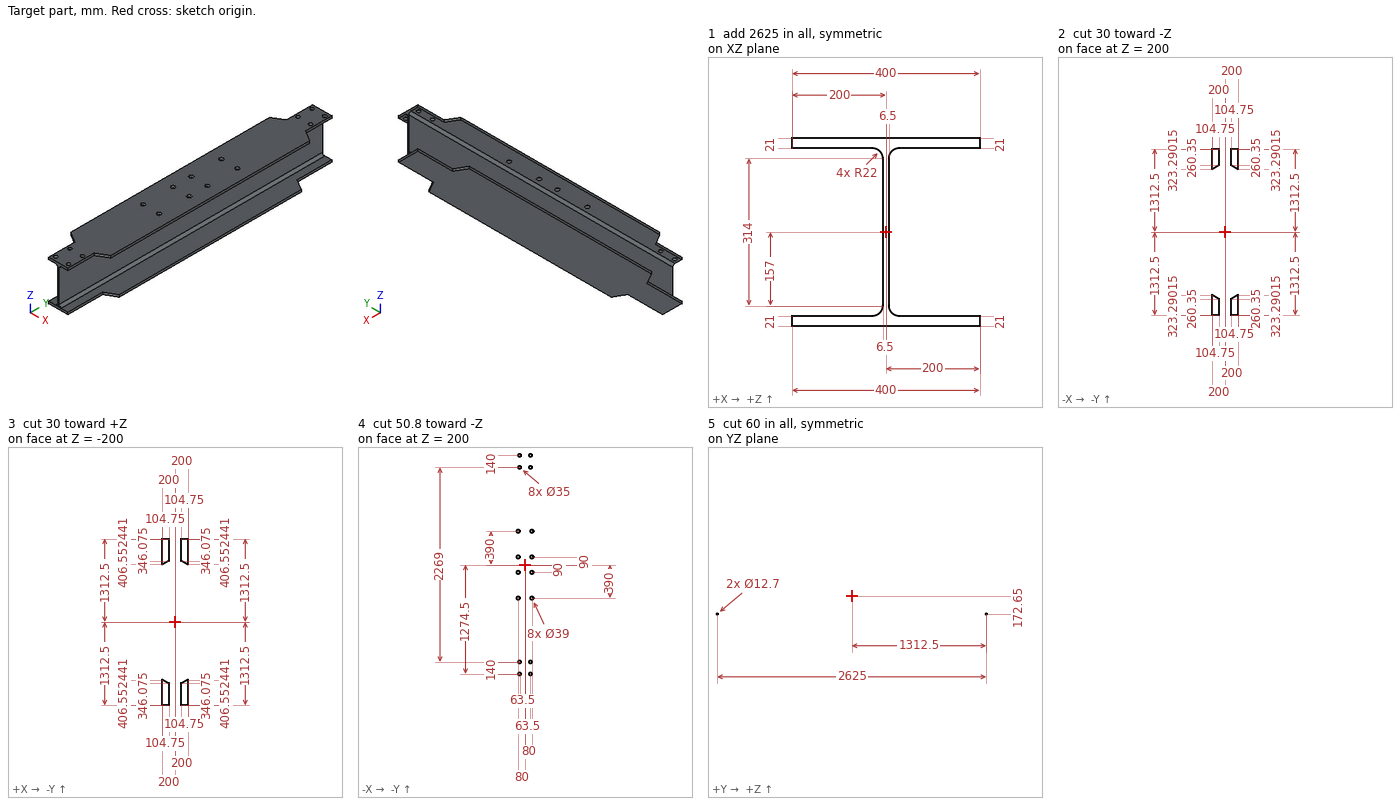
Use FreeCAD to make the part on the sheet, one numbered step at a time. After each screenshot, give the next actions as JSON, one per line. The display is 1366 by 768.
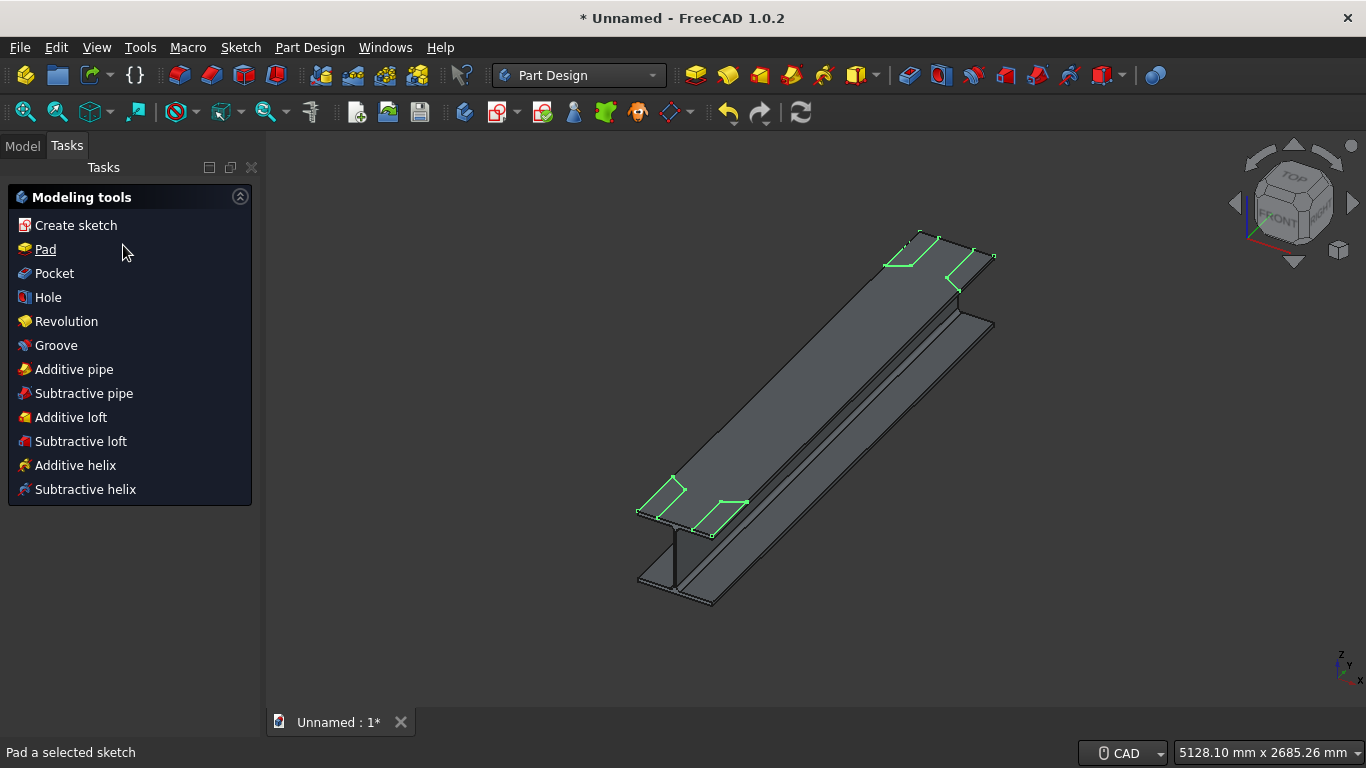
{"action": "left_click", "coordinate": [910, 76]}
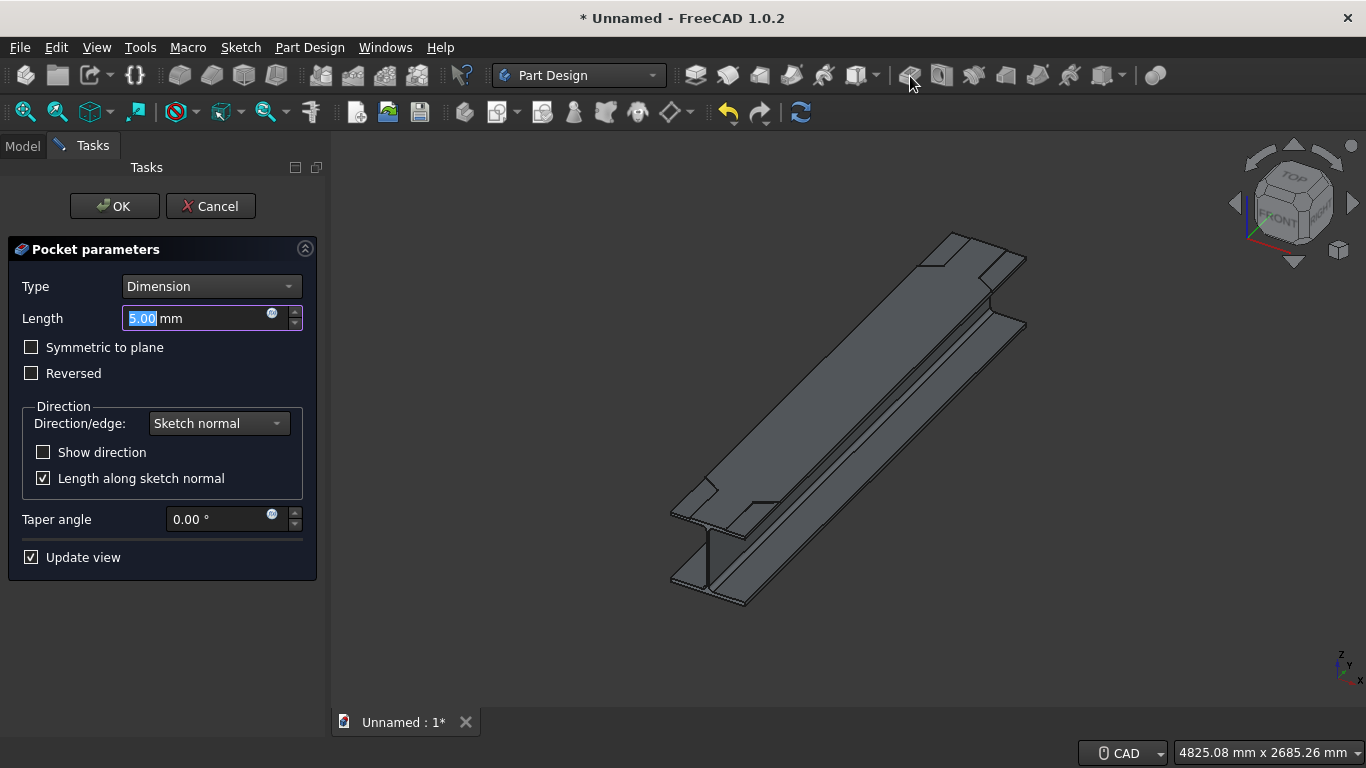
{"action": "type", "text": "30"}
{"action": "key", "text": "Tab"}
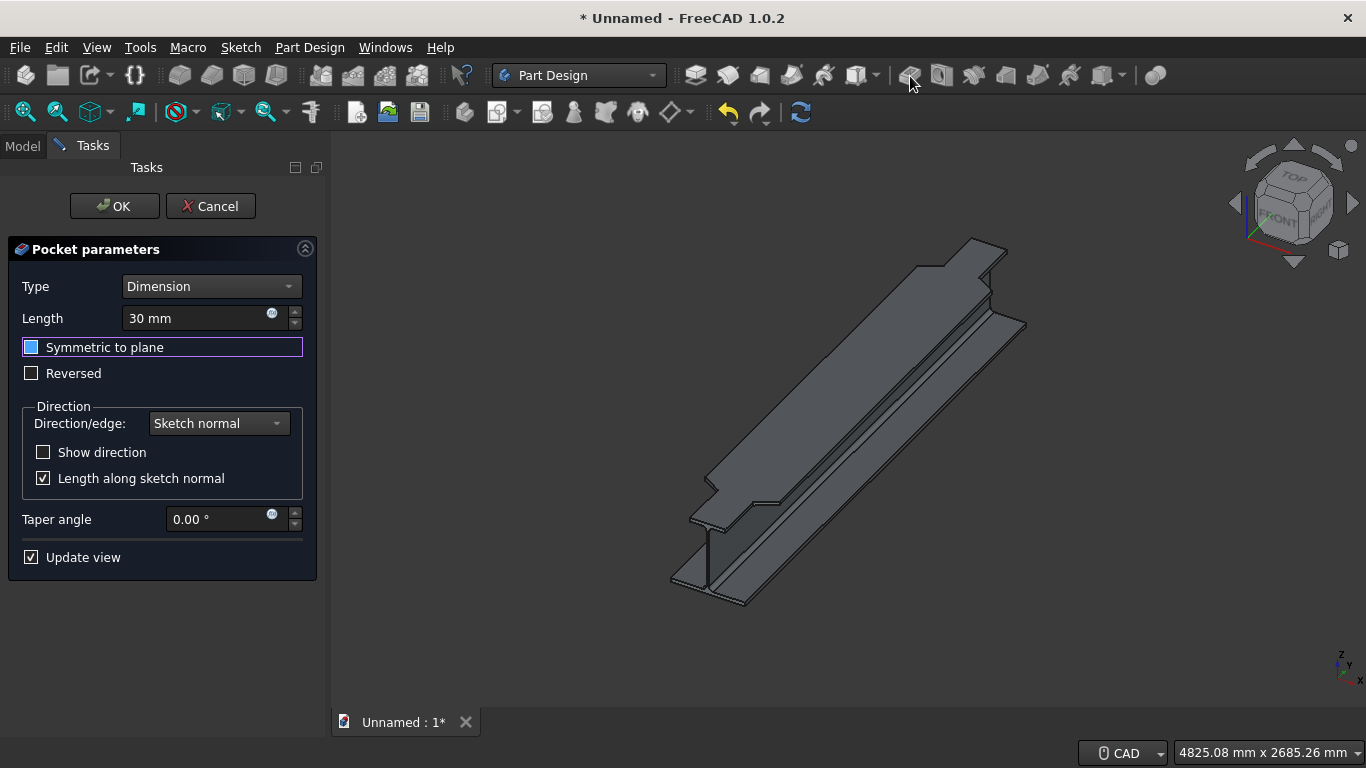
{"action": "left_click", "coordinate": [115, 206]}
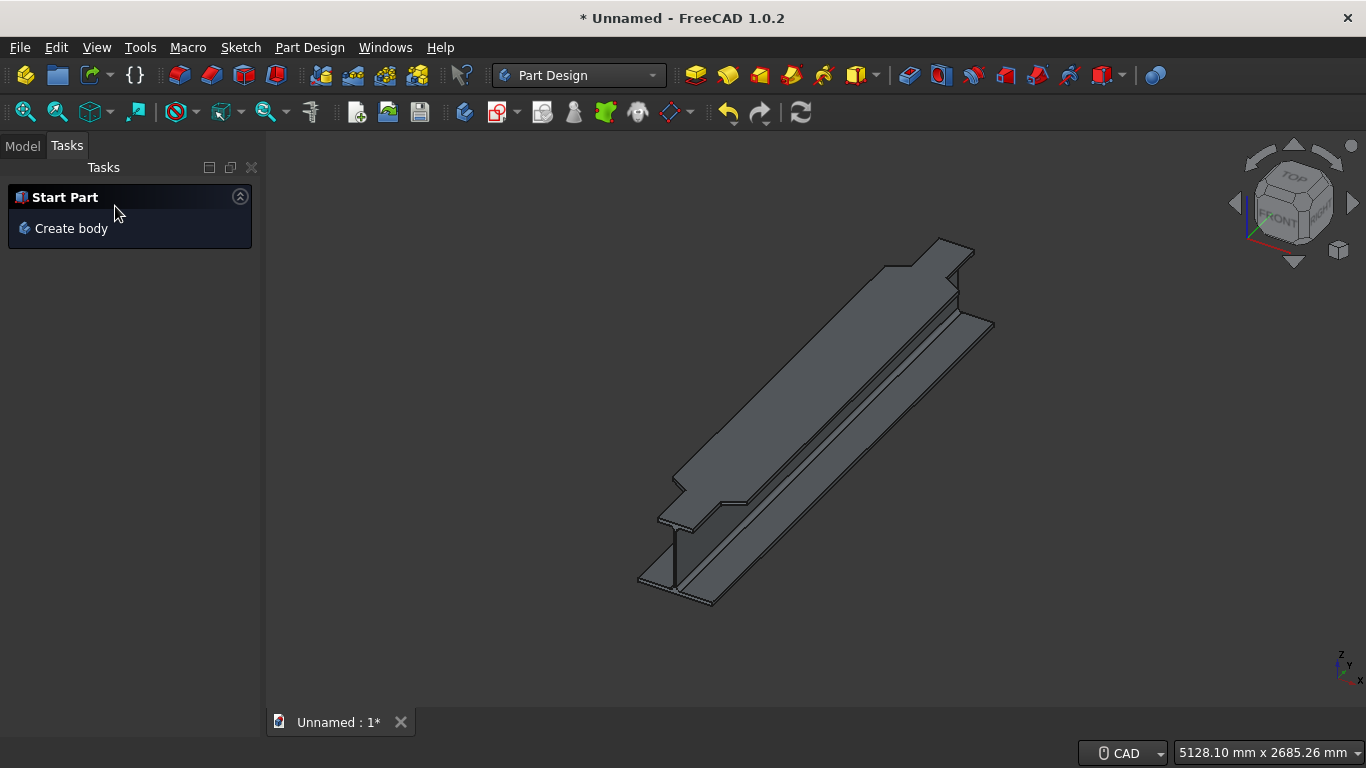
{"action": "key", "text": "5"}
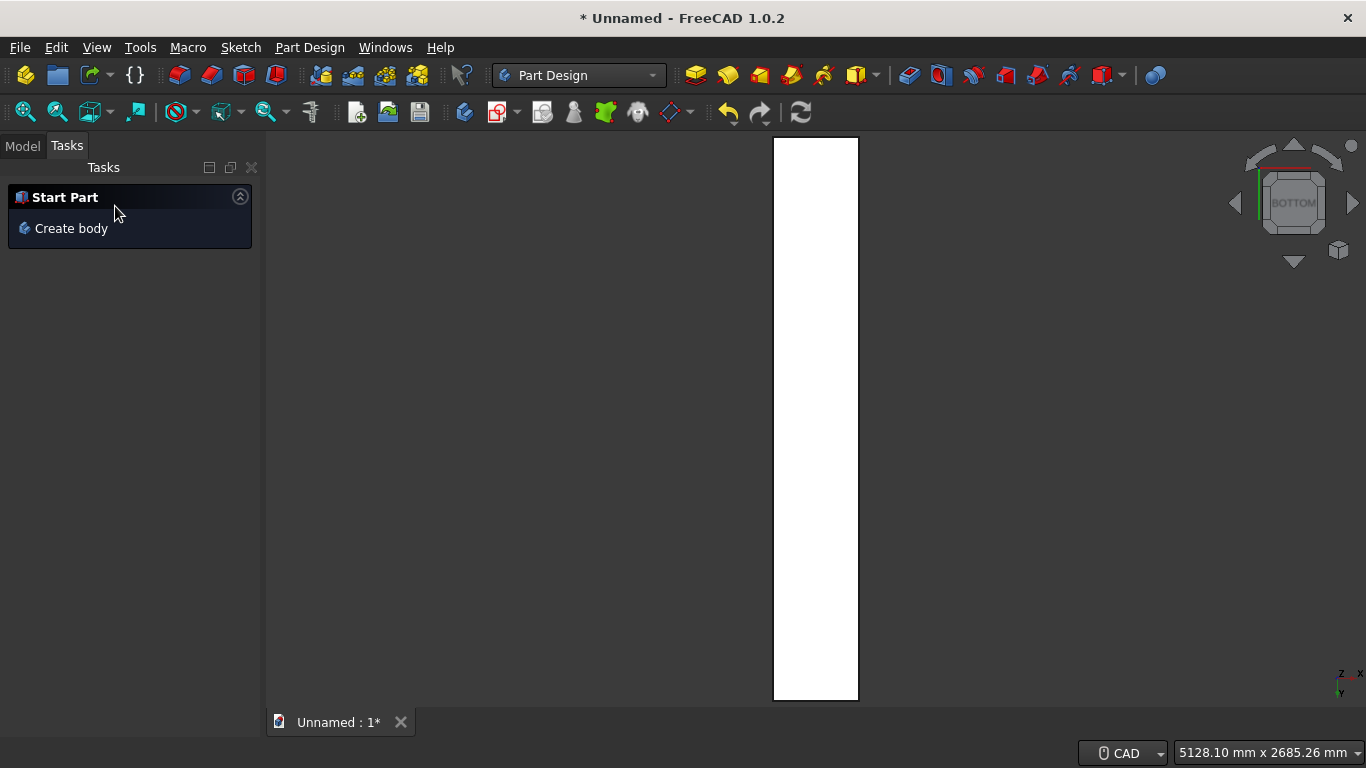
{"action": "left_click", "coordinate": [816, 579]}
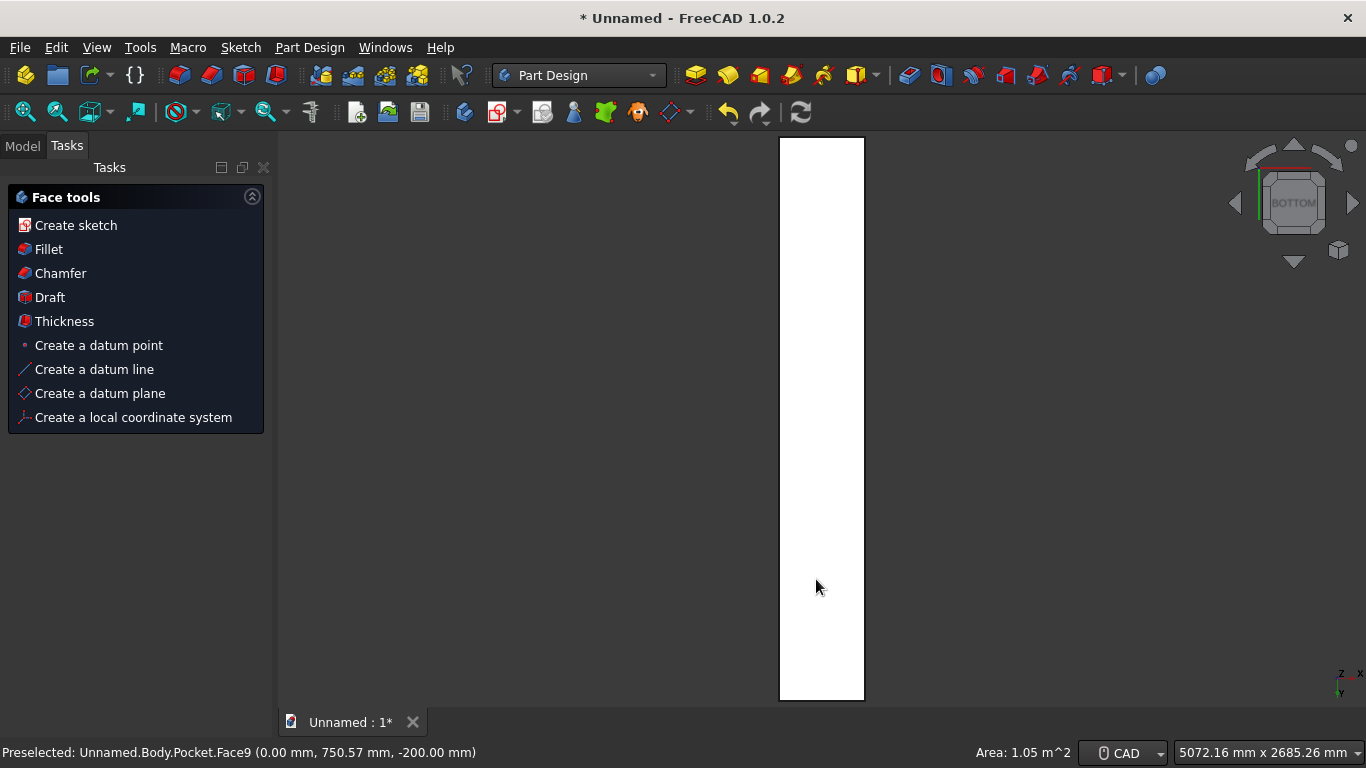
{"action": "left_click", "coordinate": [498, 112]}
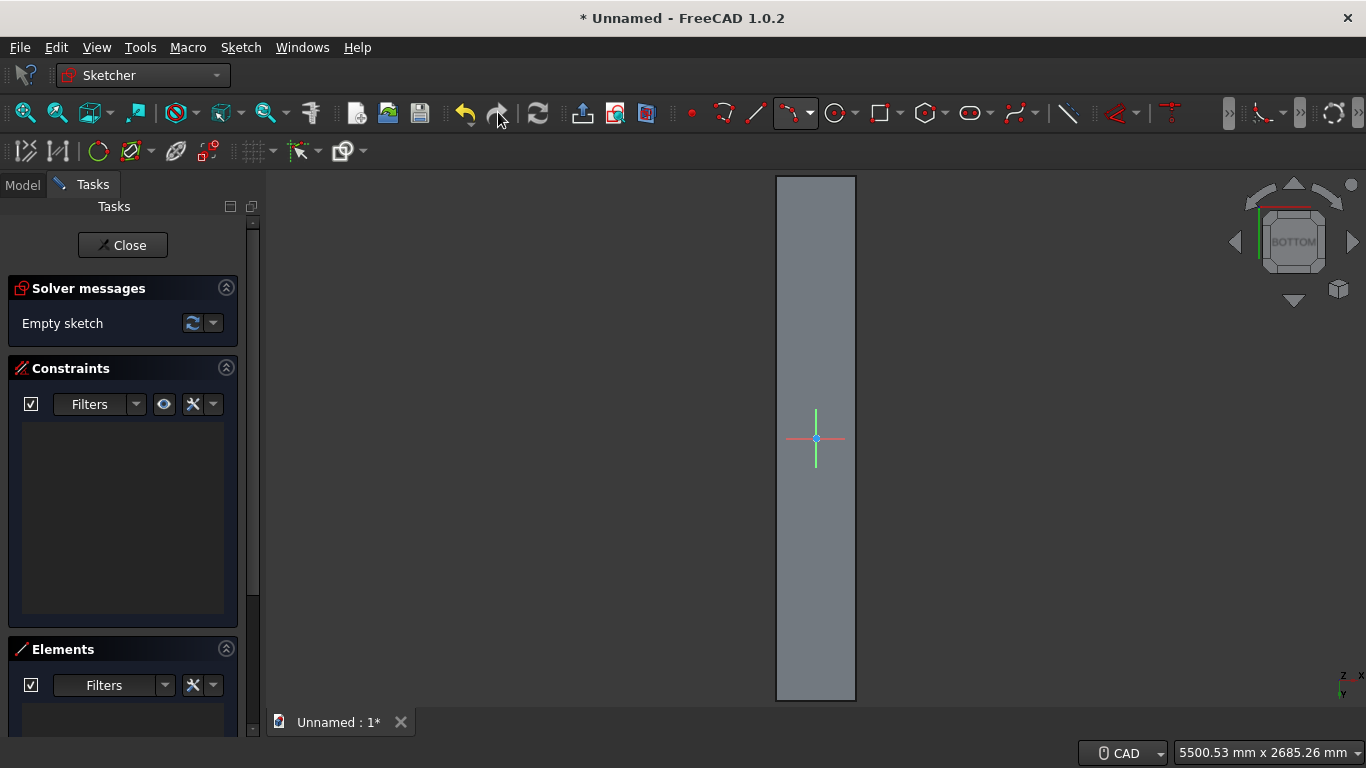
{"action": "scroll", "coordinate": [608, 439], "scroll_direction": "down", "scroll_amount": 2}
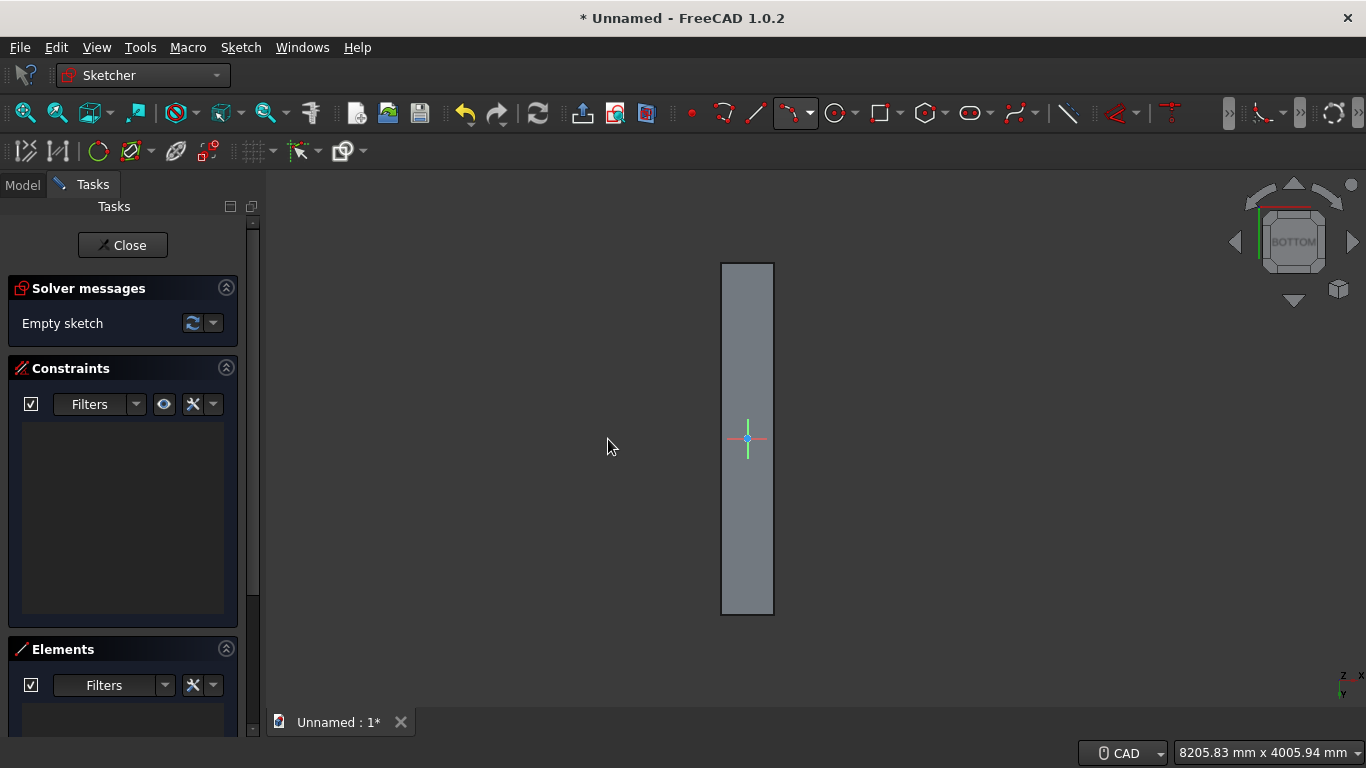
{"action": "left_click", "coordinate": [724, 114]}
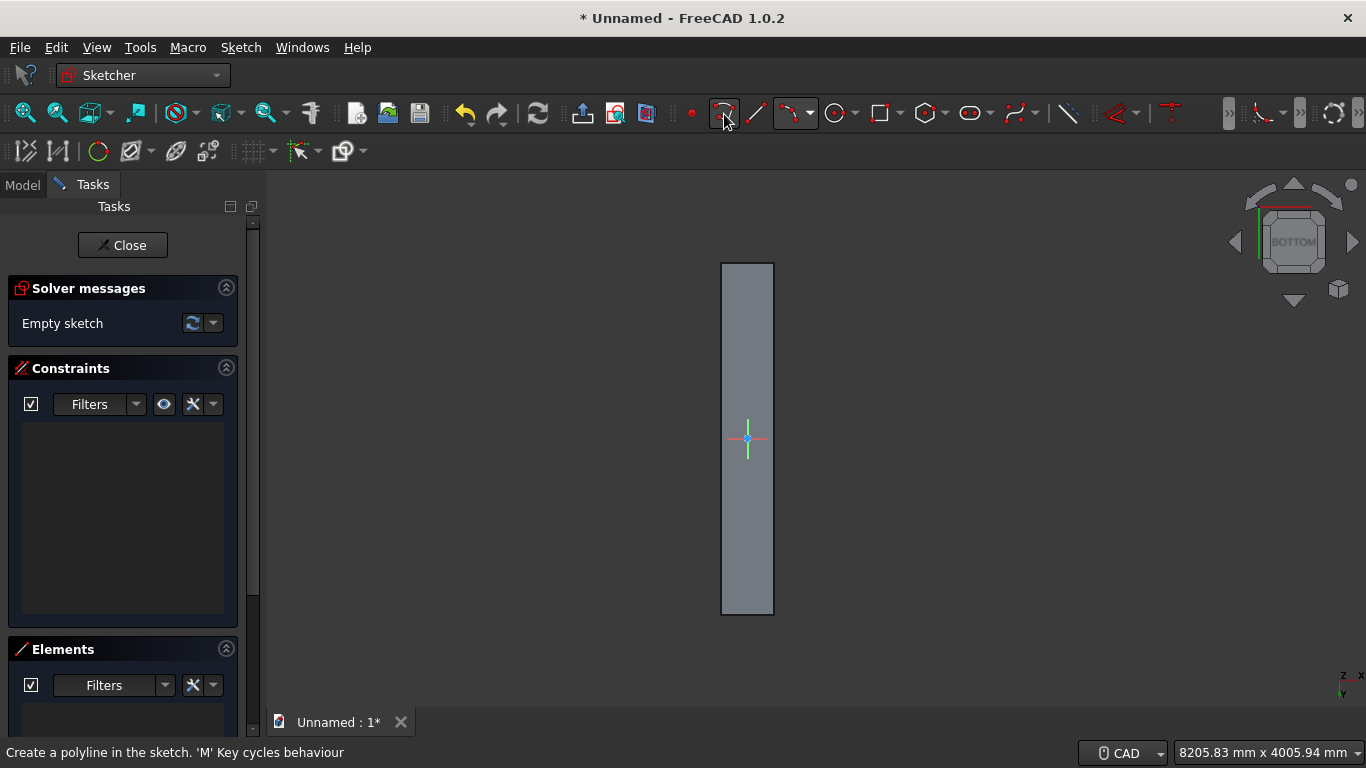
{"action": "left_click", "coordinate": [774, 560]}